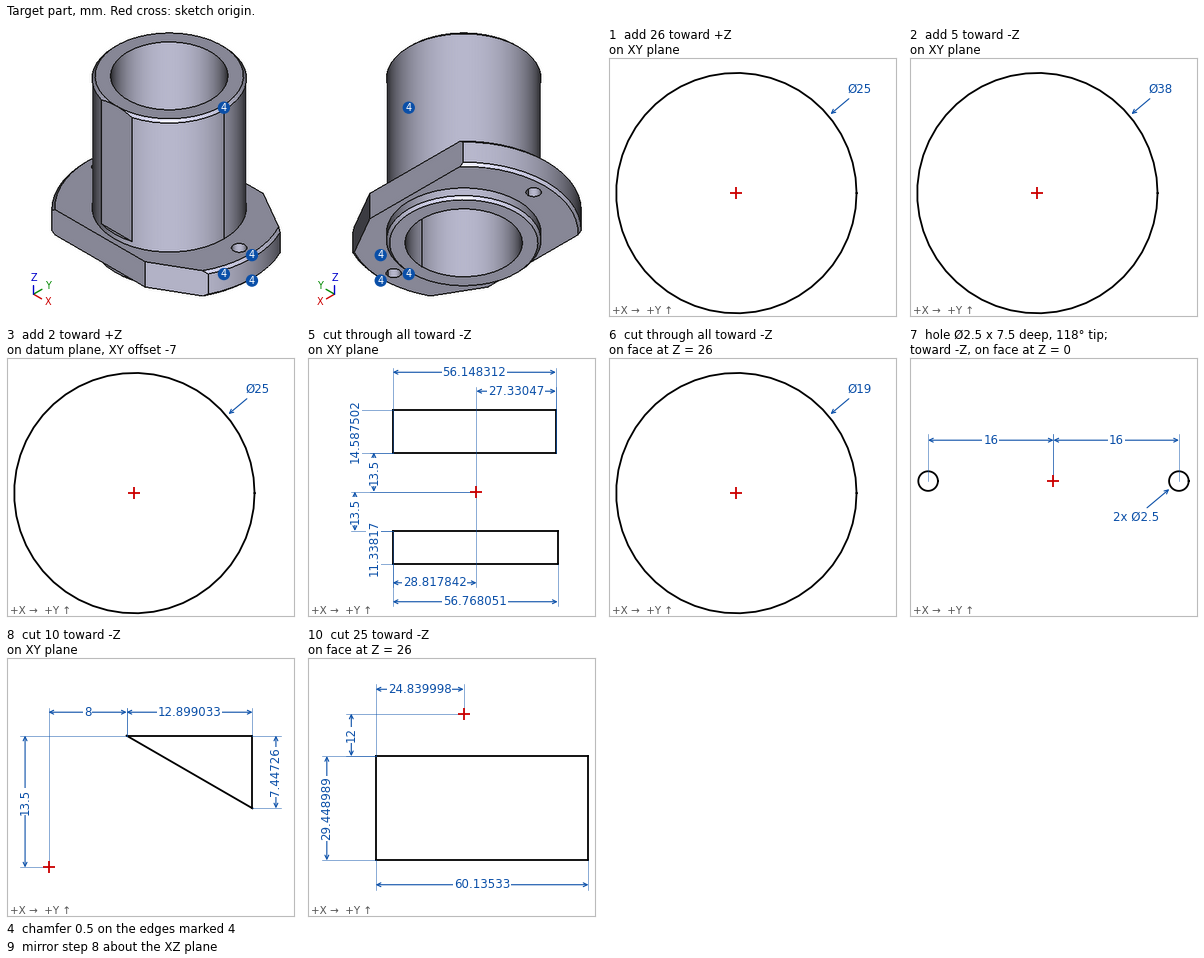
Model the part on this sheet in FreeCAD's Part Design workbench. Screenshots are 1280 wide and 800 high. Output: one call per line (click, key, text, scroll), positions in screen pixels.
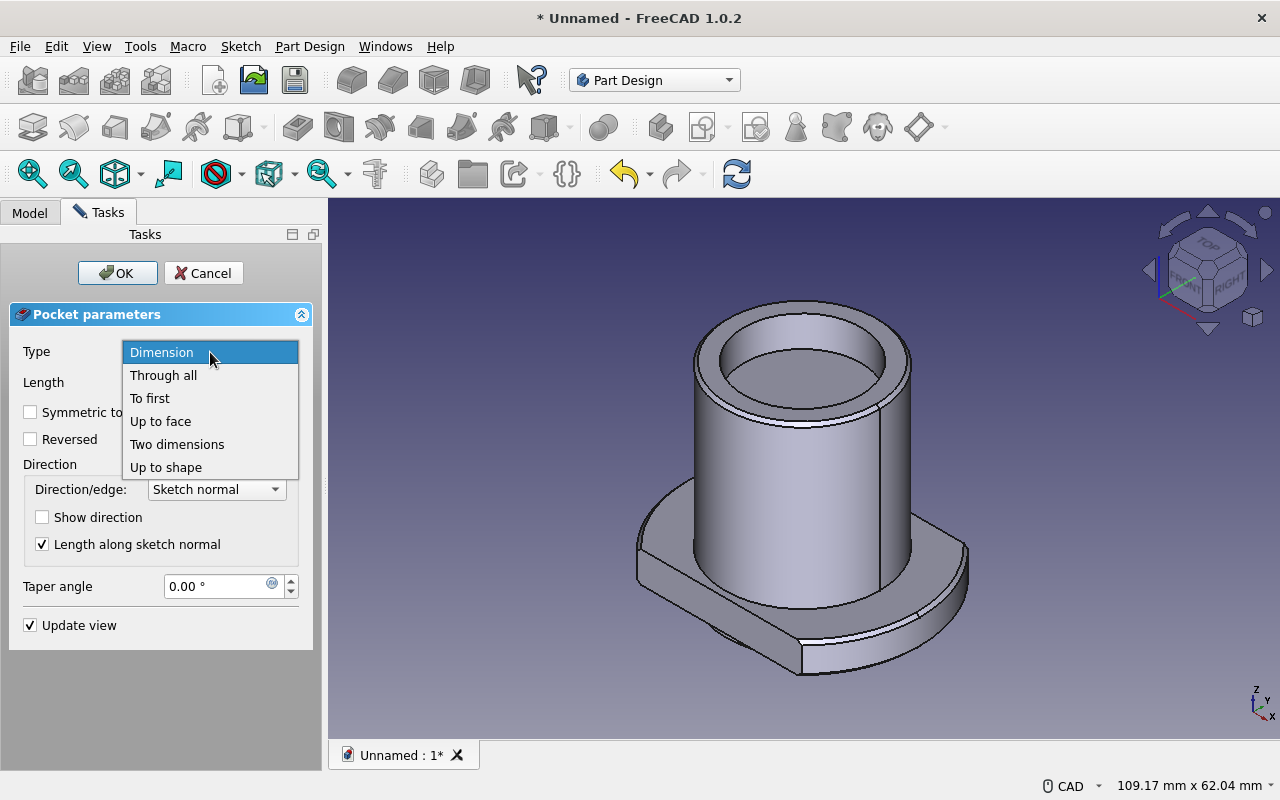
click(208, 376)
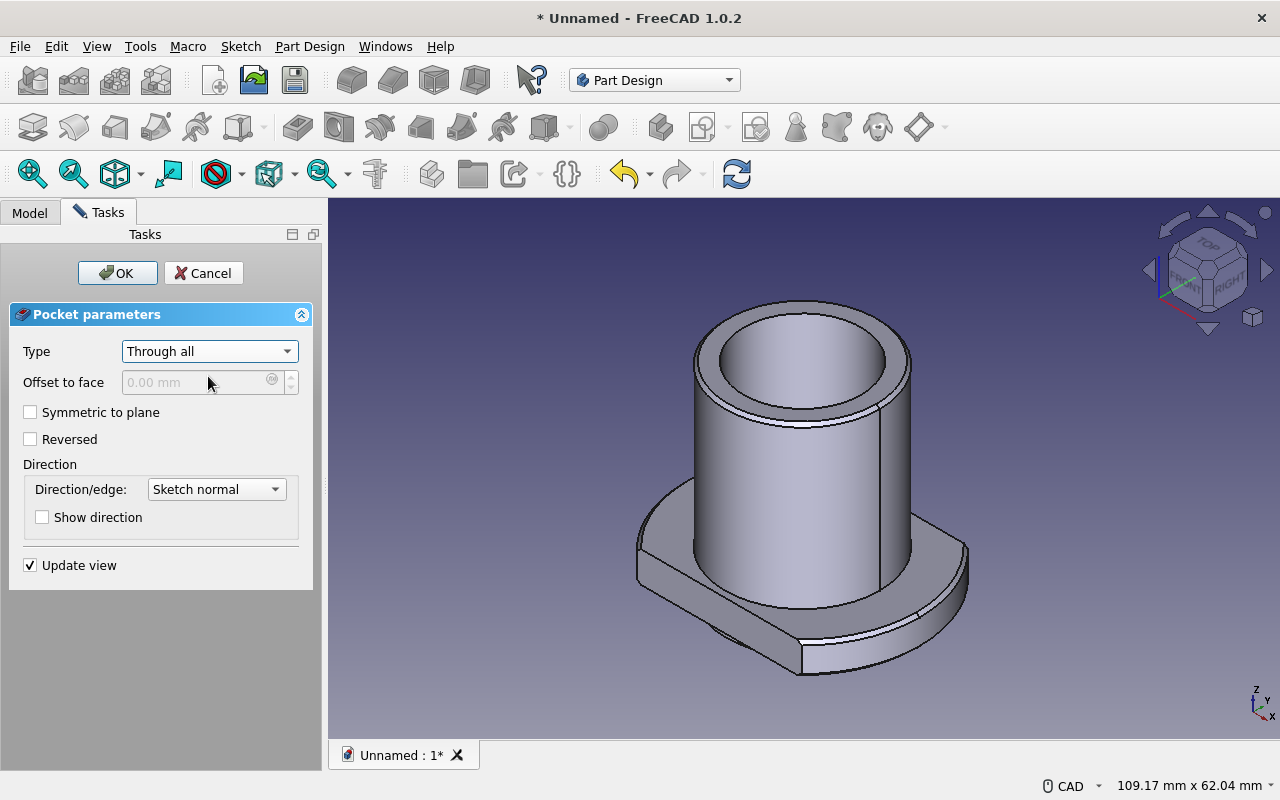
click(118, 273)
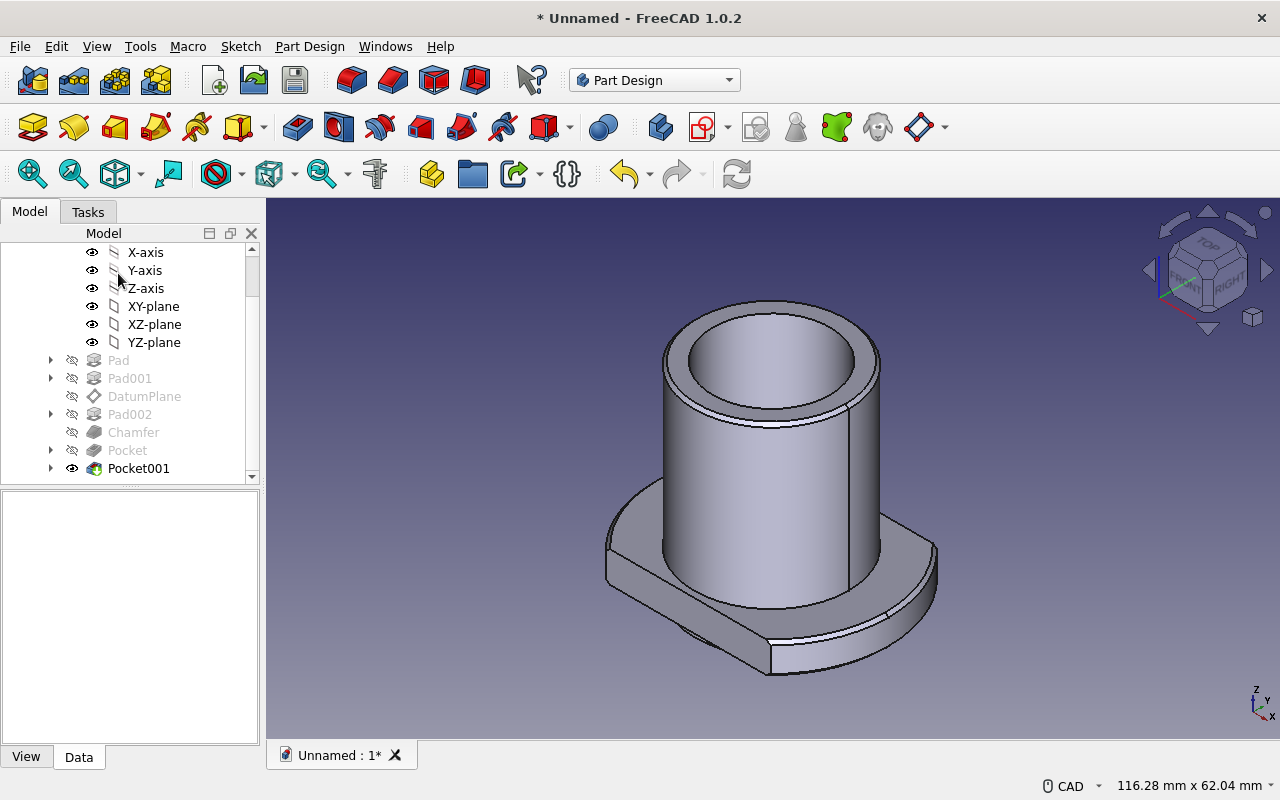
click(869, 602)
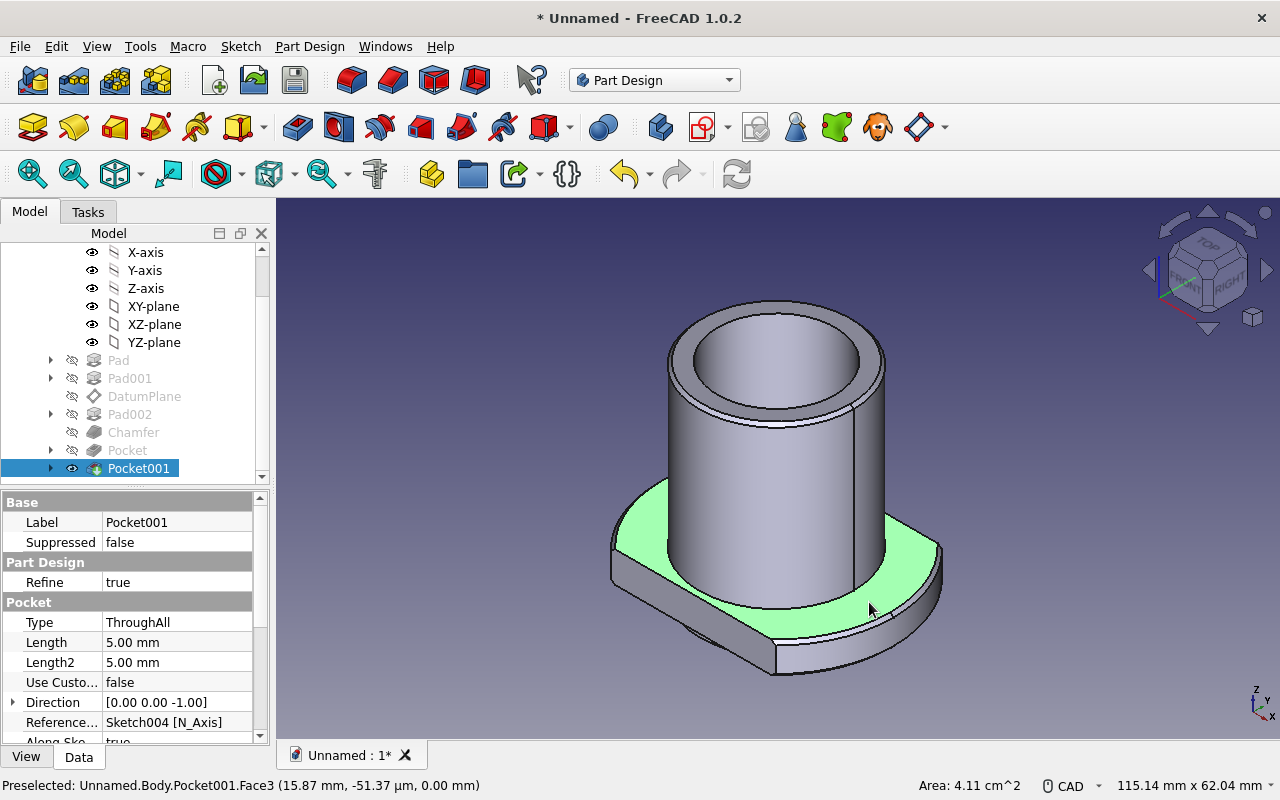
click(702, 128)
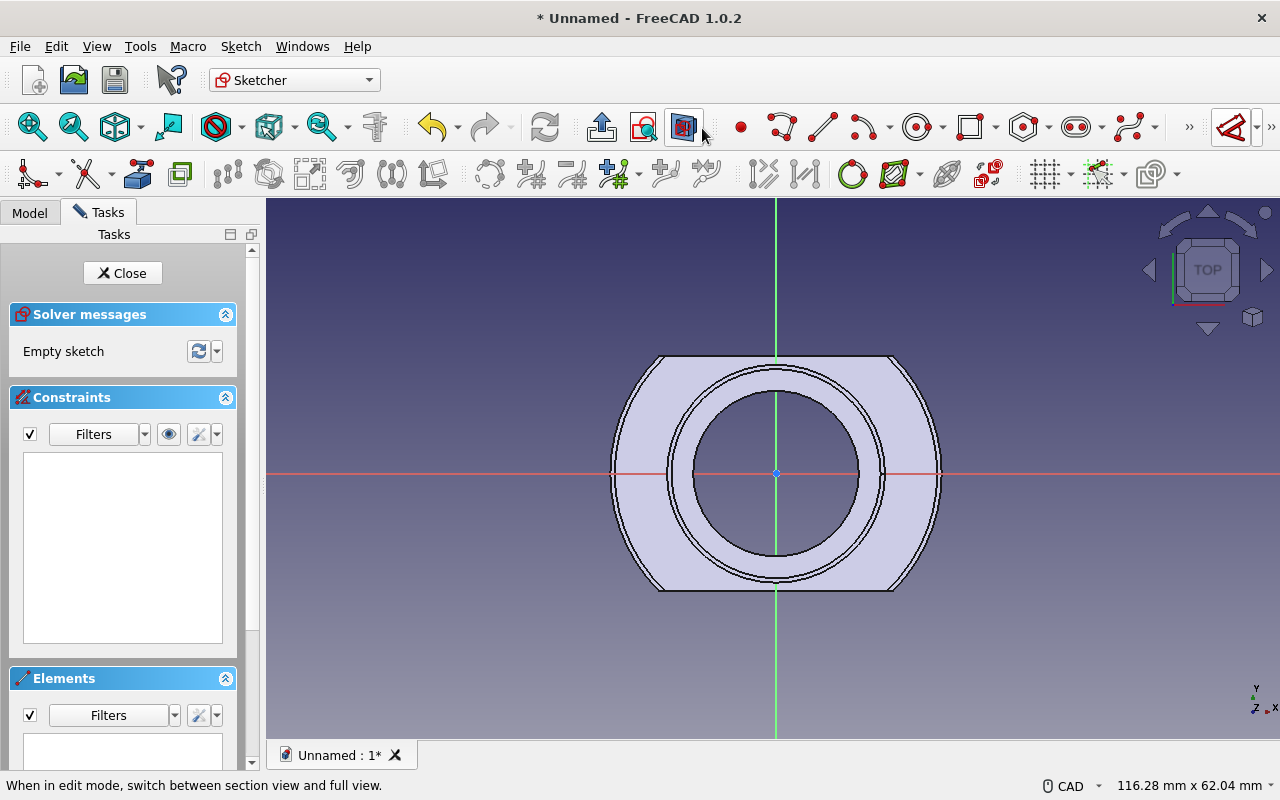
click(684, 128)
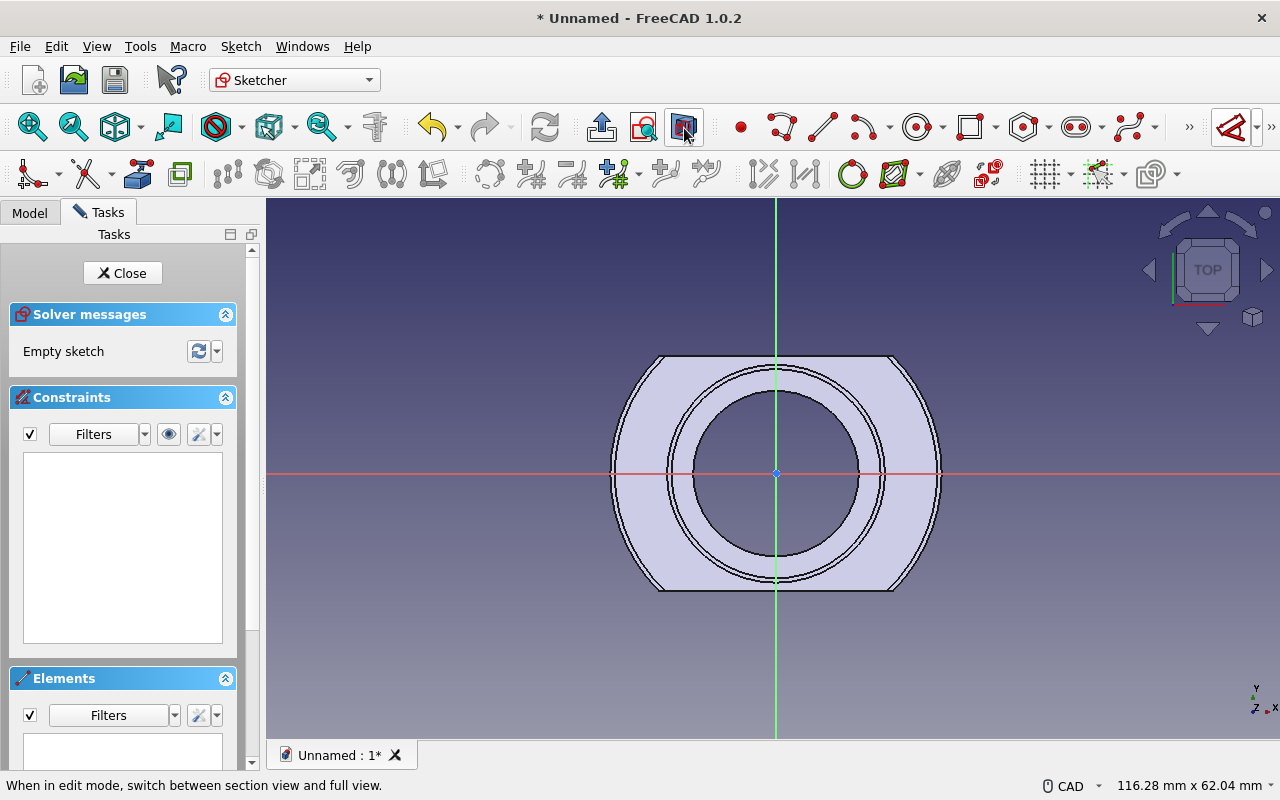
scroll(863, 480, up, 3)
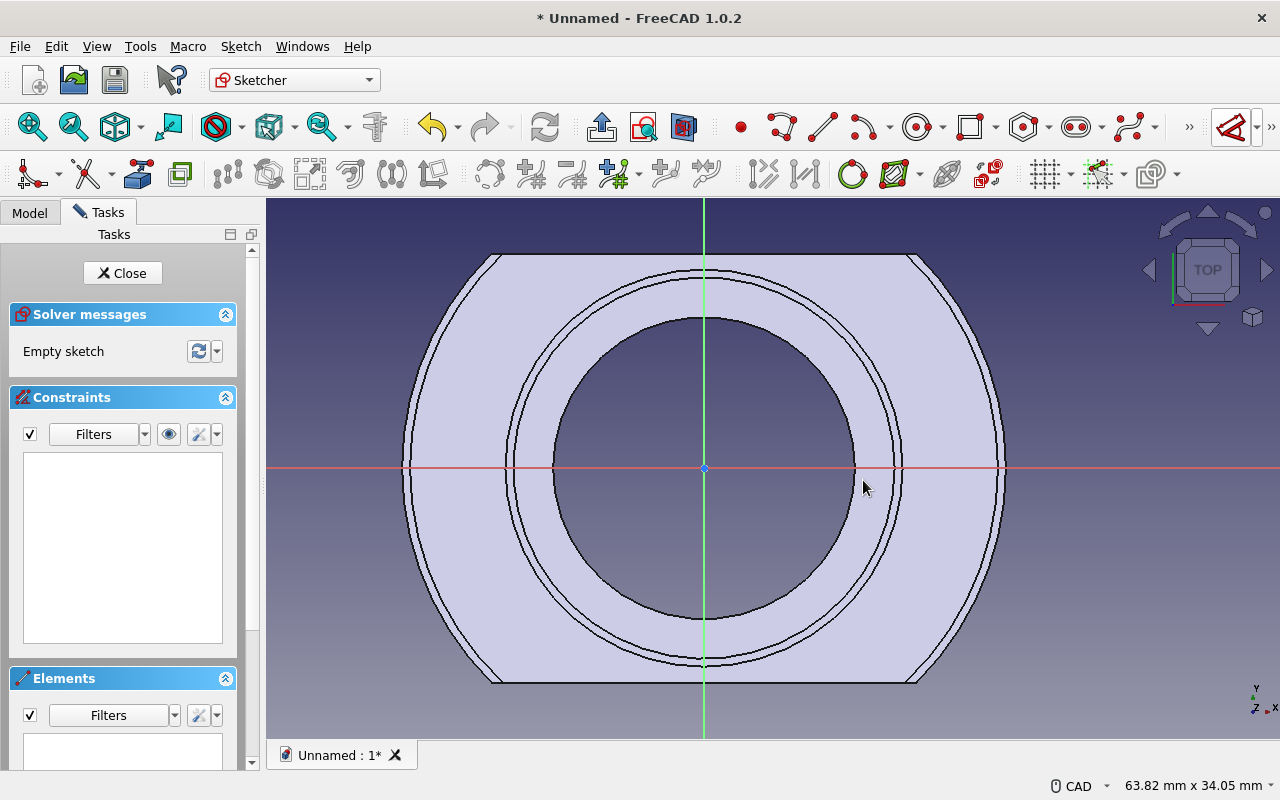
click(916, 128)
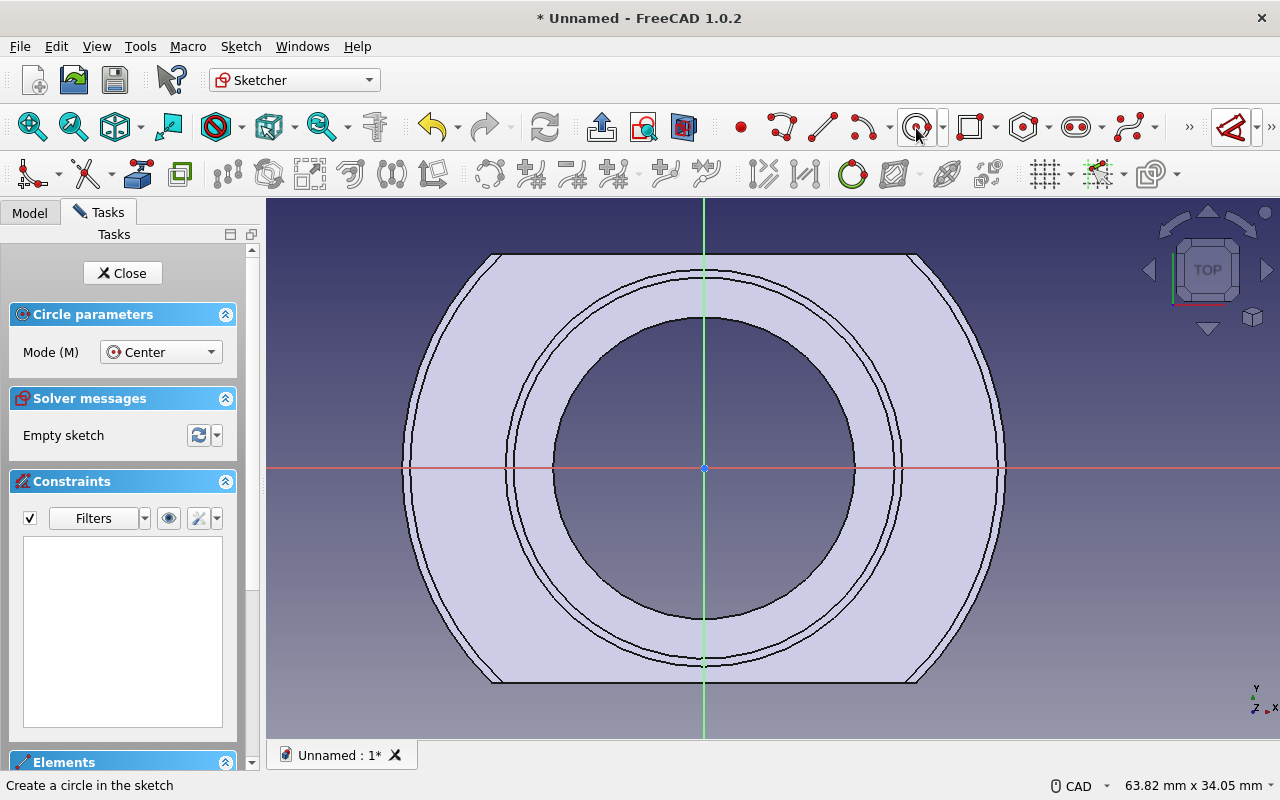
click(958, 468)
click(972, 454)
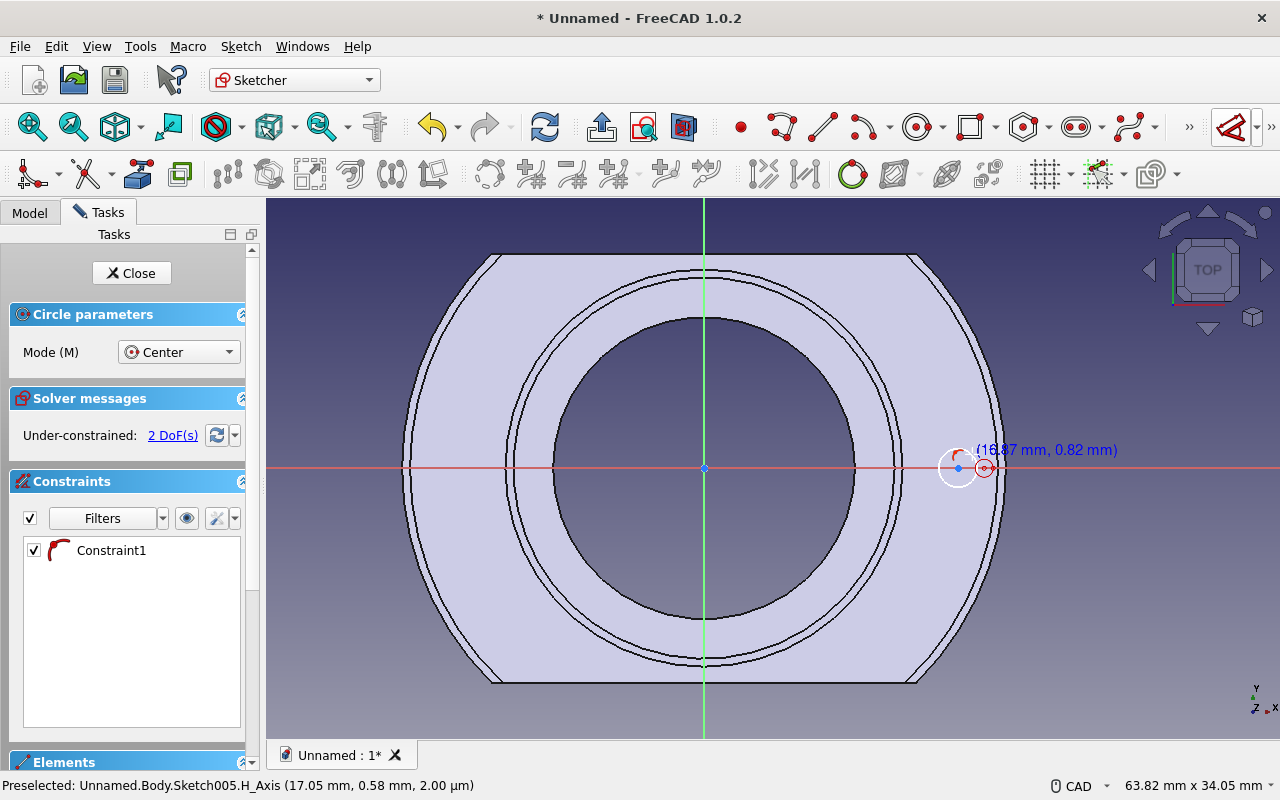
click(450, 468)
click(464, 454)
key(Escape)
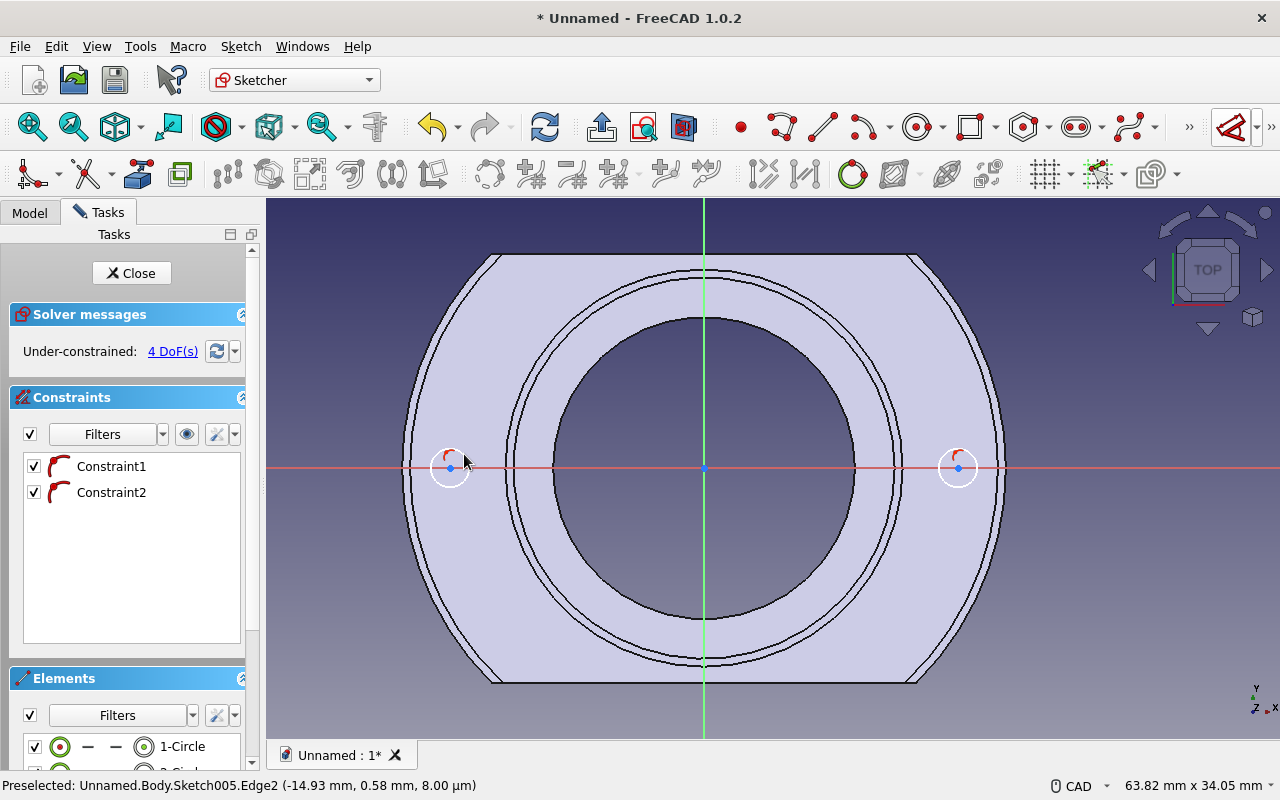
click(972, 455)